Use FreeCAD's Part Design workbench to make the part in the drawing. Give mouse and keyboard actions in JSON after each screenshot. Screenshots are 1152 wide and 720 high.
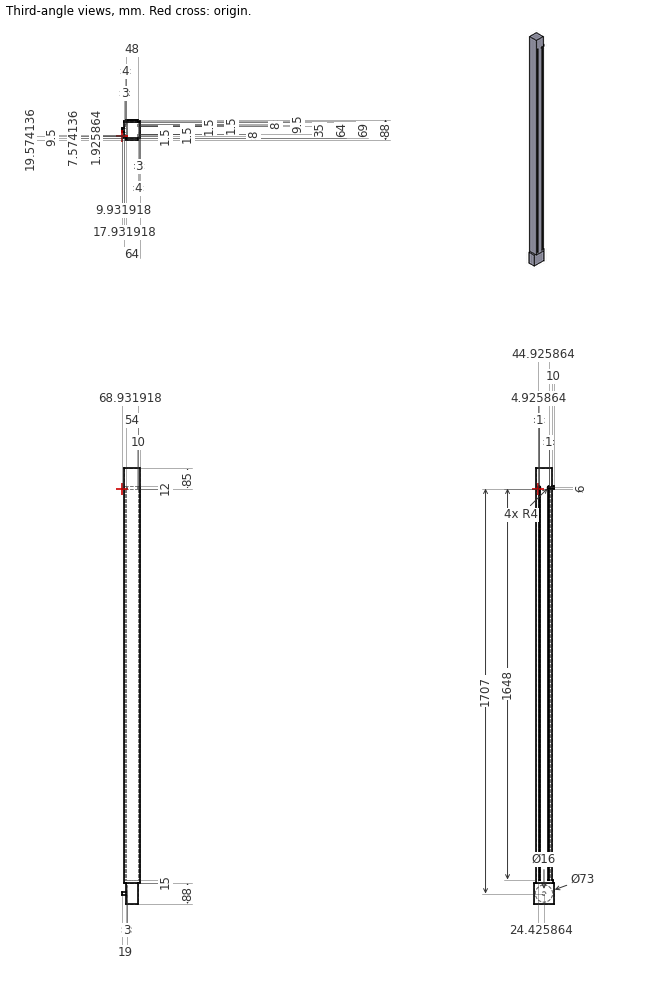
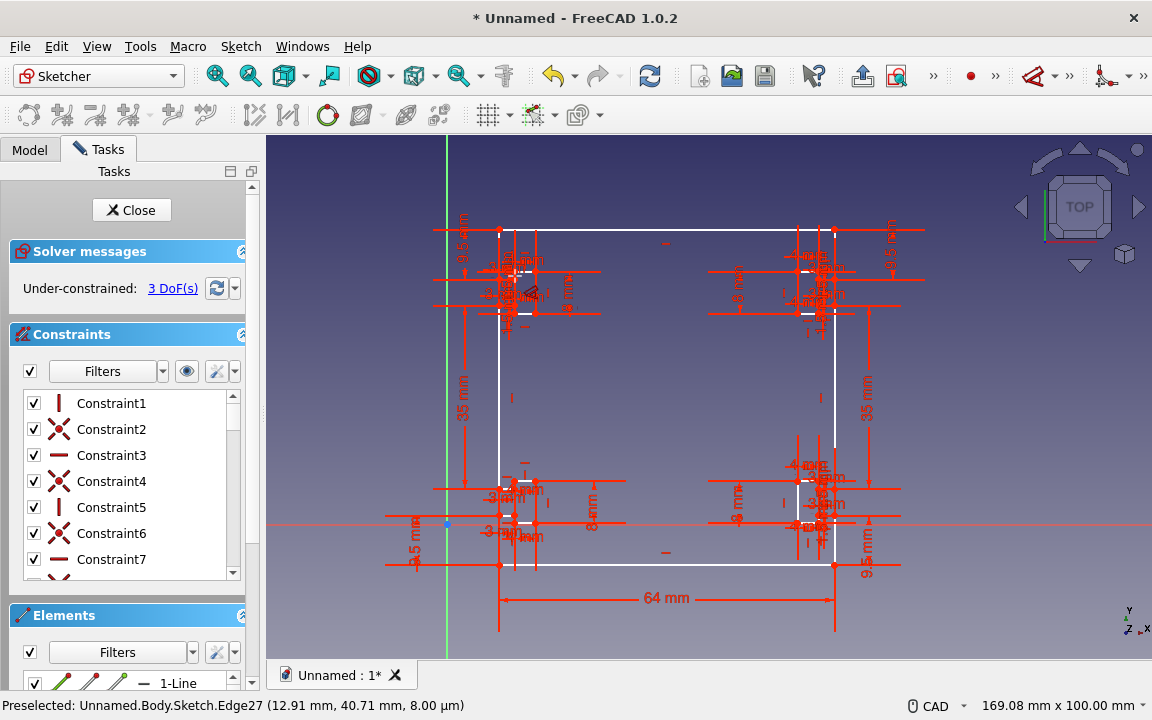
{"action": "scroll", "coordinate": [515, 487], "scroll_direction": "up", "scroll_amount": 9}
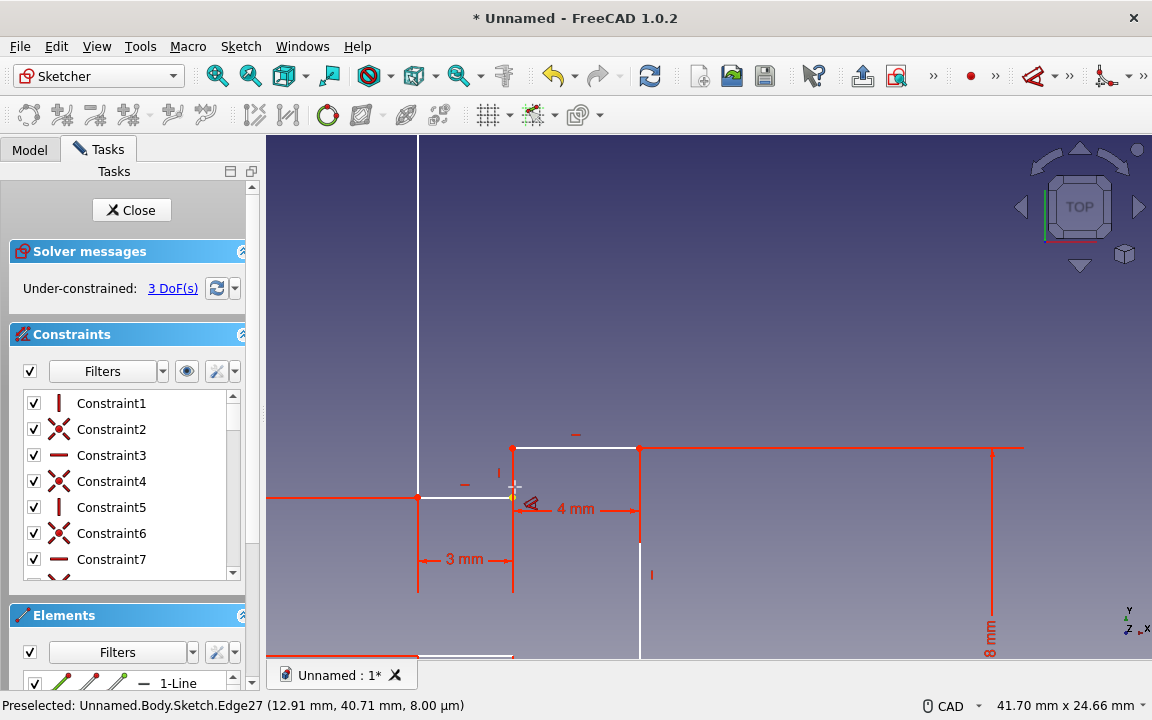
{"action": "left_click", "coordinate": [513, 483]}
{"action": "left_click", "coordinate": [479, 473]}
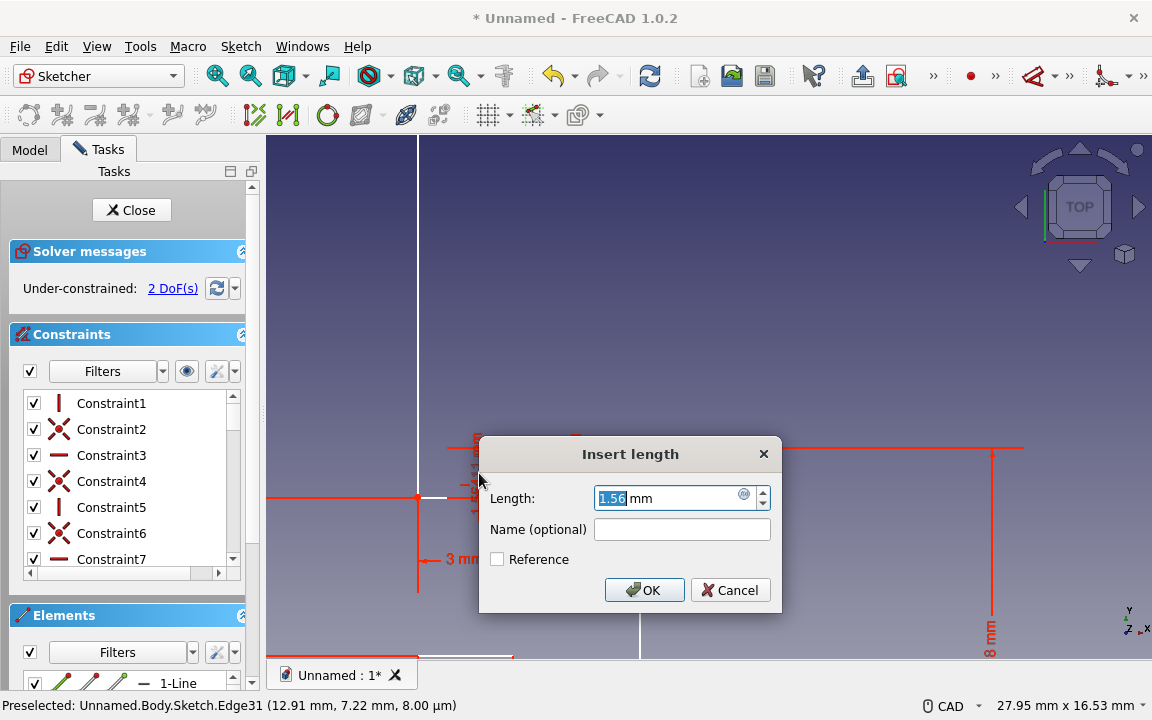
{"action": "type", "text": "1.5"}
{"action": "key", "text": "Return"}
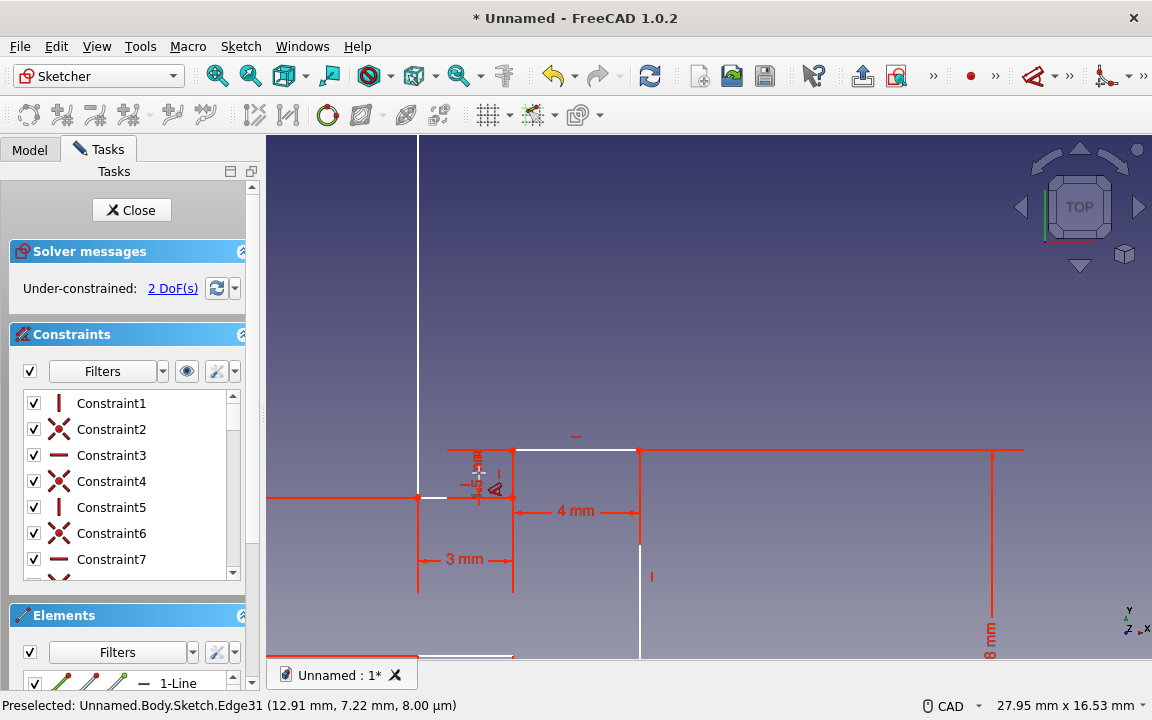
{"action": "scroll", "coordinate": [515, 488], "scroll_direction": "down", "scroll_amount": 9}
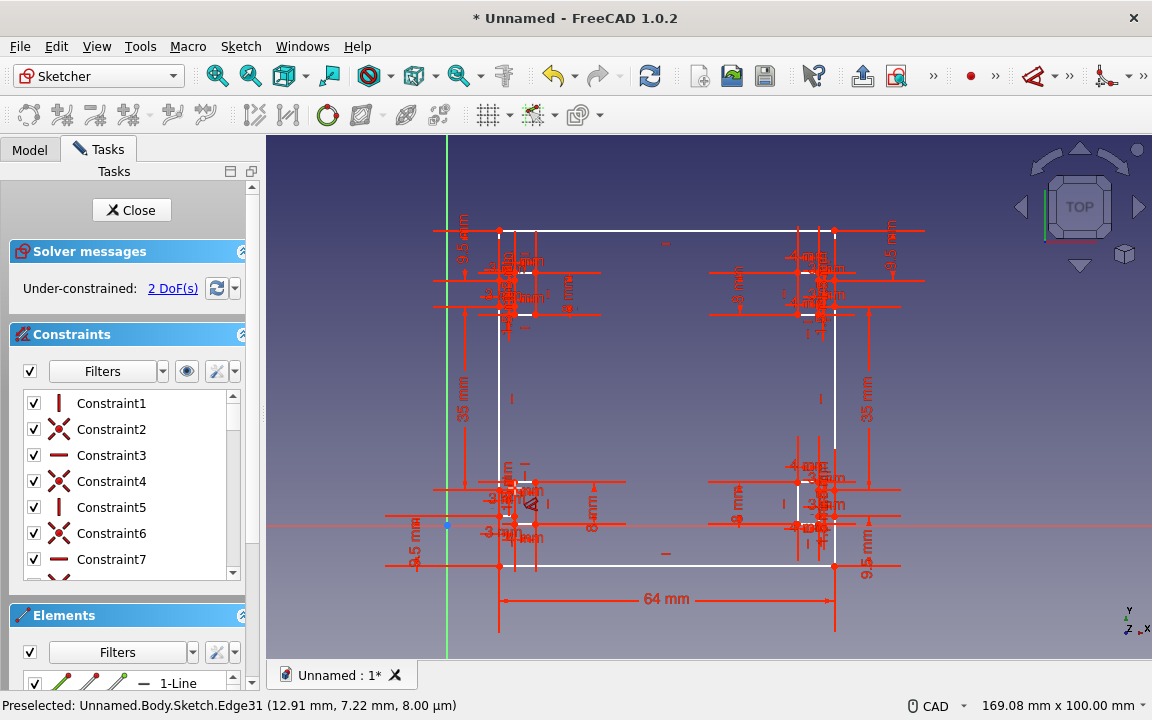
{"action": "left_click", "coordinate": [499, 516]}
{"action": "left_click", "coordinate": [473, 584]}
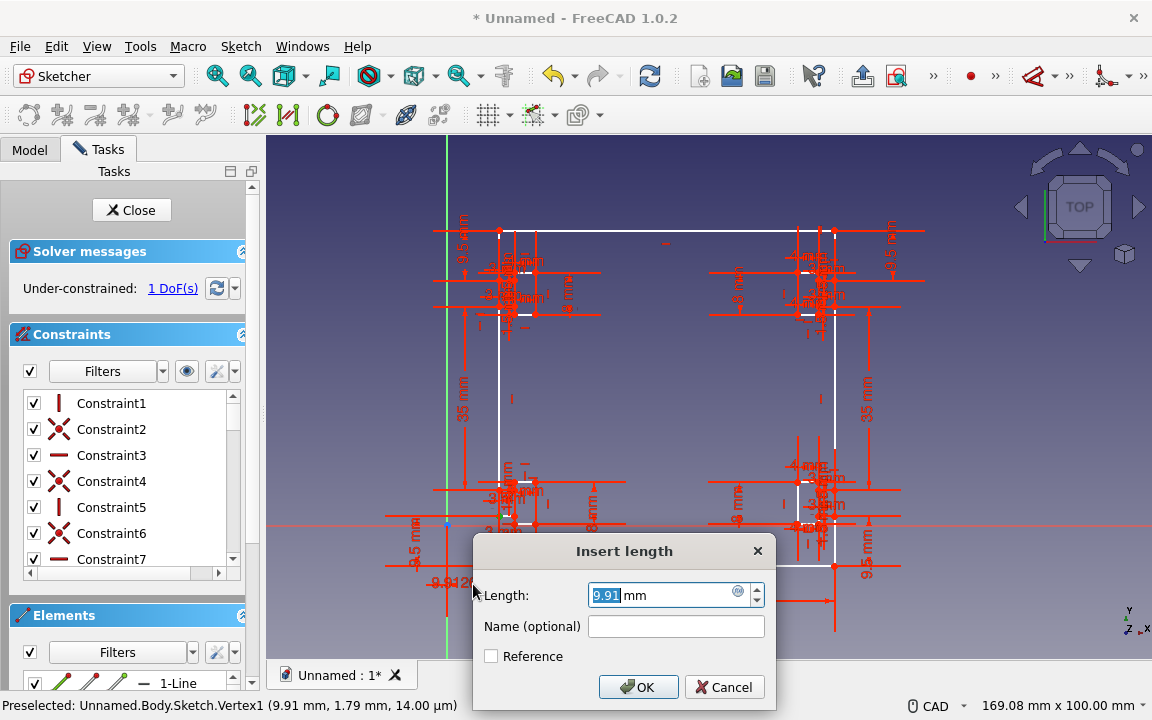
{"action": "type", "text": "9.931918"}
{"action": "key", "text": "Return"}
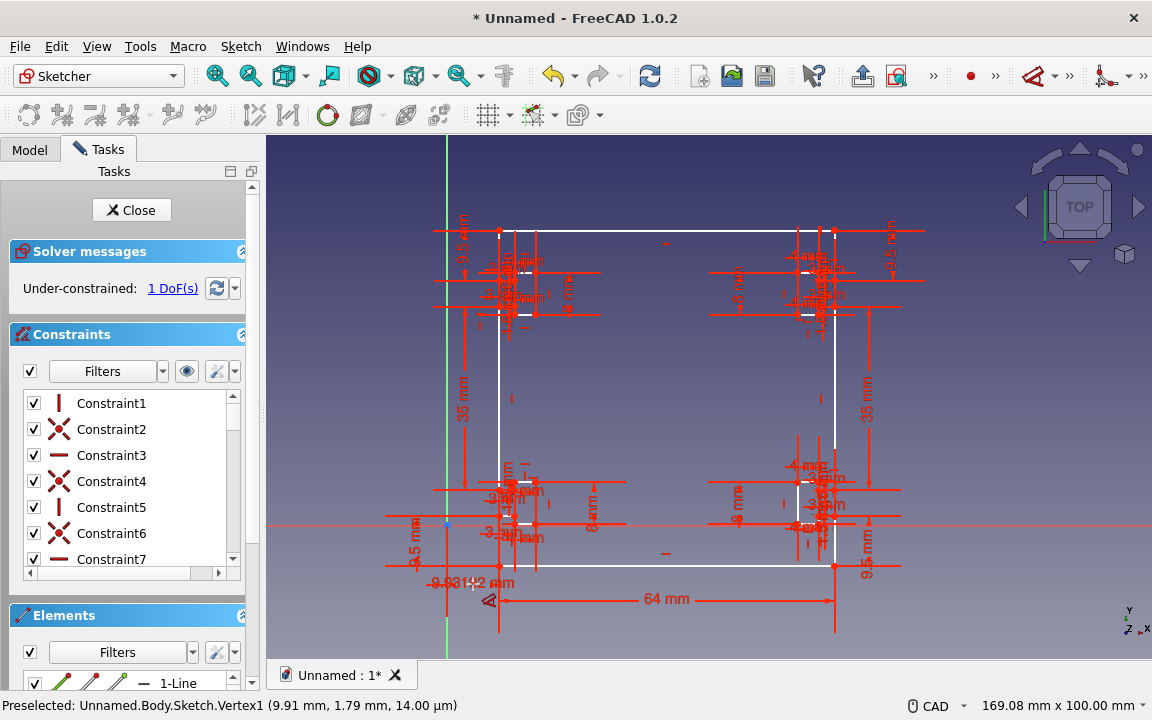
{"action": "scroll", "coordinate": [499, 516], "scroll_direction": "up", "scroll_amount": 7}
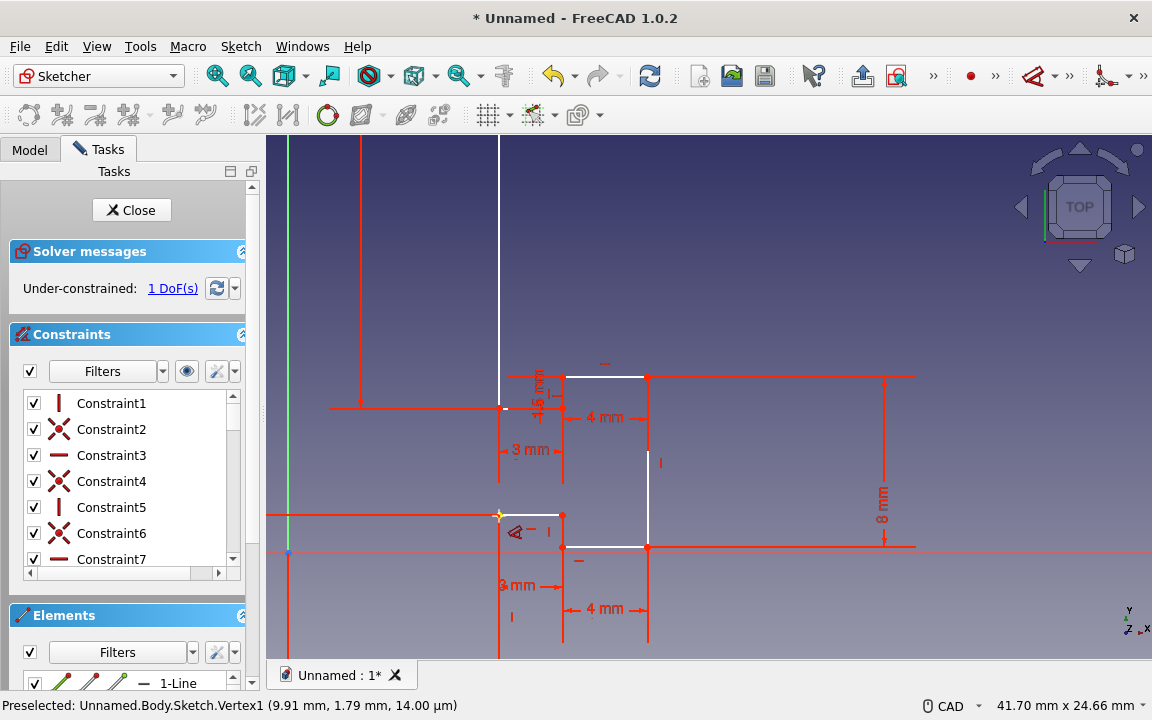
{"action": "left_click", "coordinate": [499, 515]}
{"action": "left_click", "coordinate": [533, 534]}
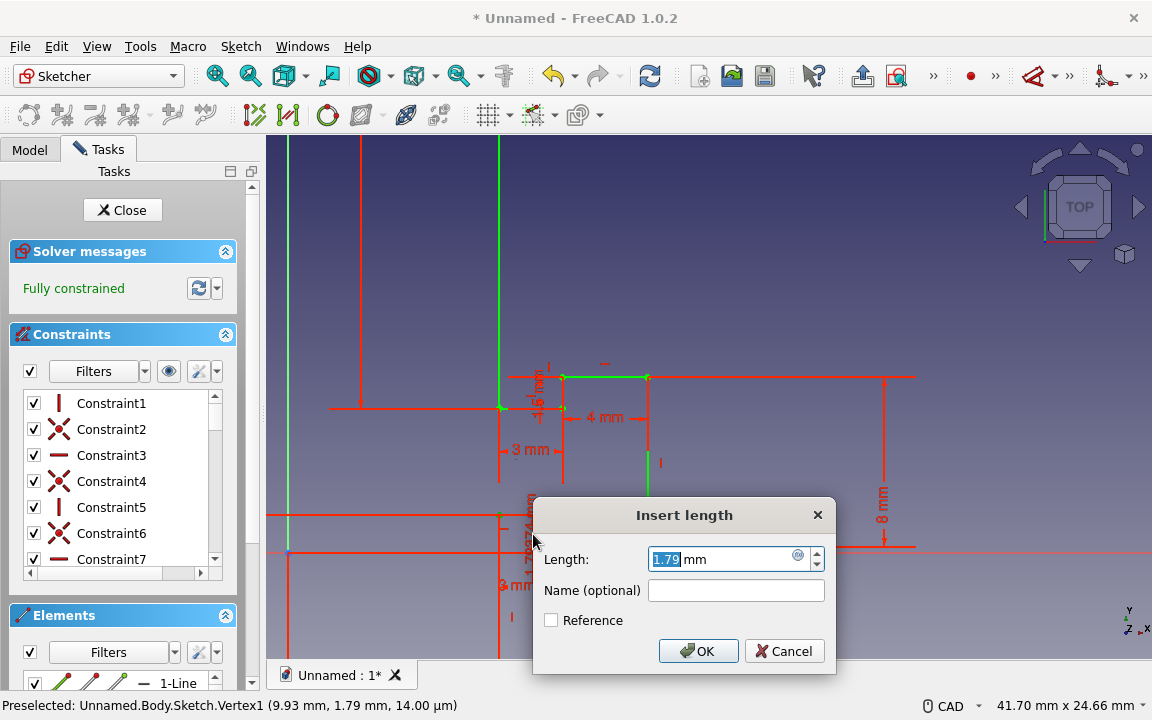
{"action": "type", "text": "1.925864"}
{"action": "key", "text": "Return"}
{"action": "key", "text": "Escape"}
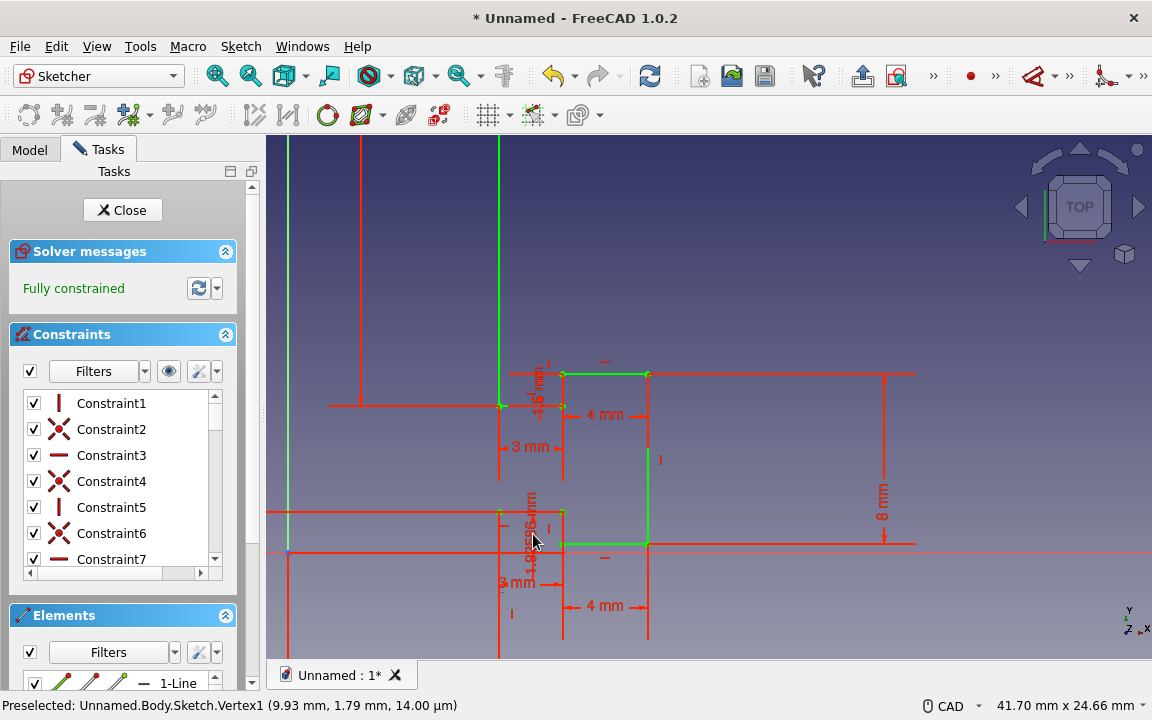
{"action": "left_click", "coordinate": [123, 210]}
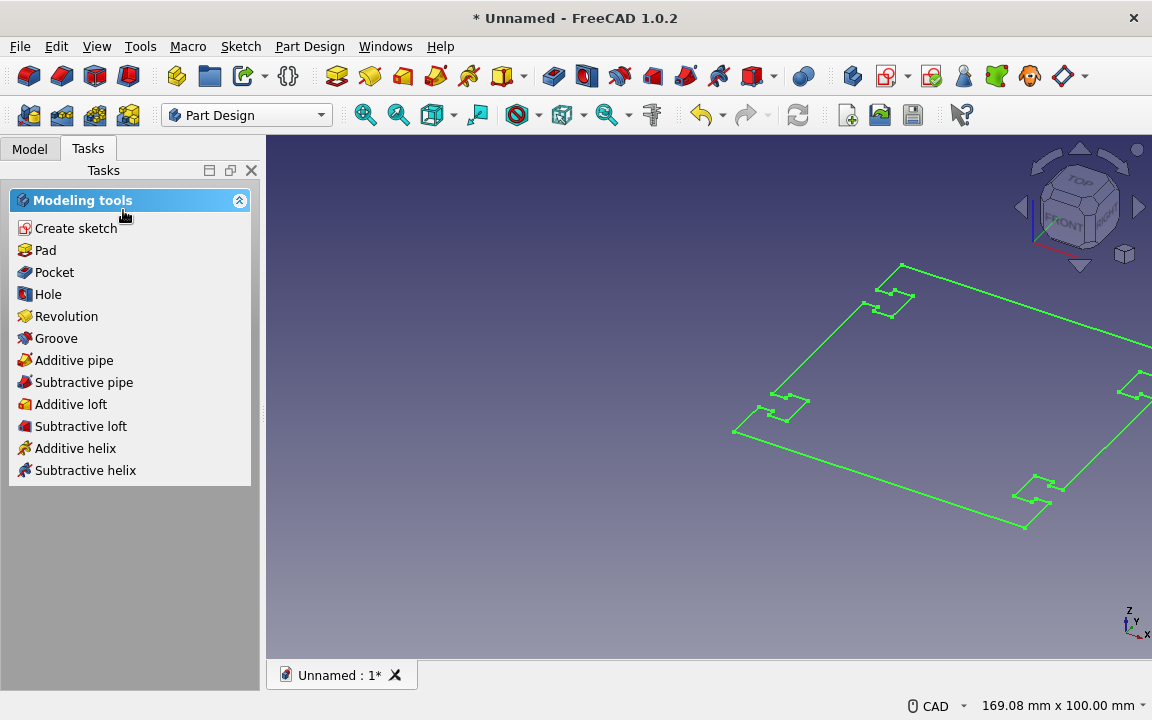
{"action": "left_click", "coordinate": [337, 76]}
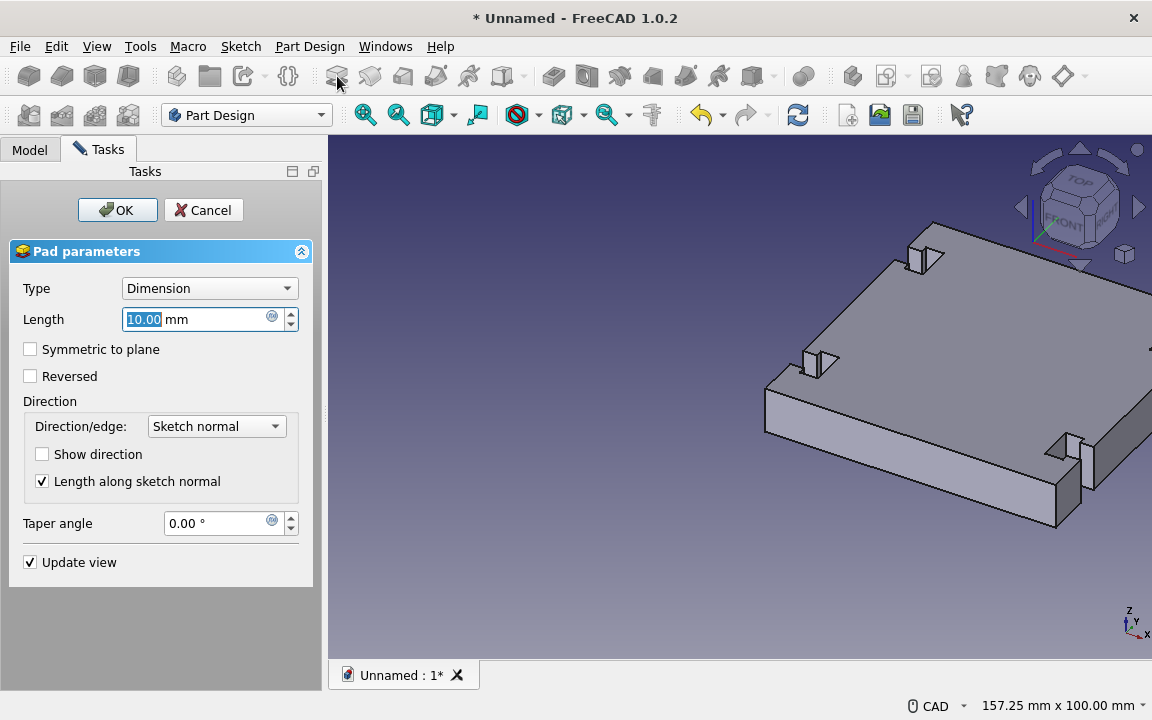
{"action": "type", "text": "1648"}
{"action": "key", "text": "Tab"}